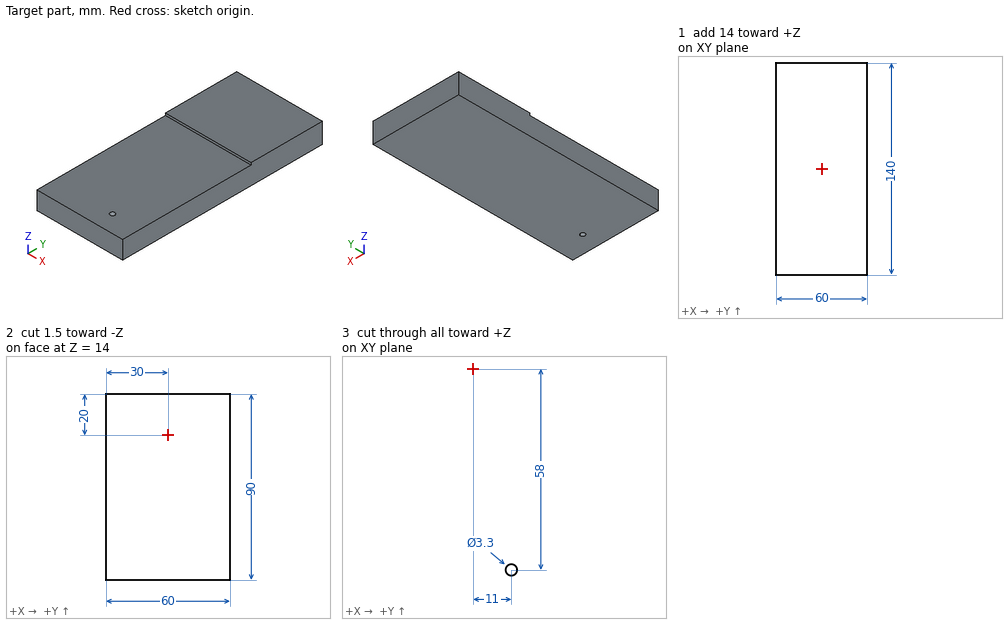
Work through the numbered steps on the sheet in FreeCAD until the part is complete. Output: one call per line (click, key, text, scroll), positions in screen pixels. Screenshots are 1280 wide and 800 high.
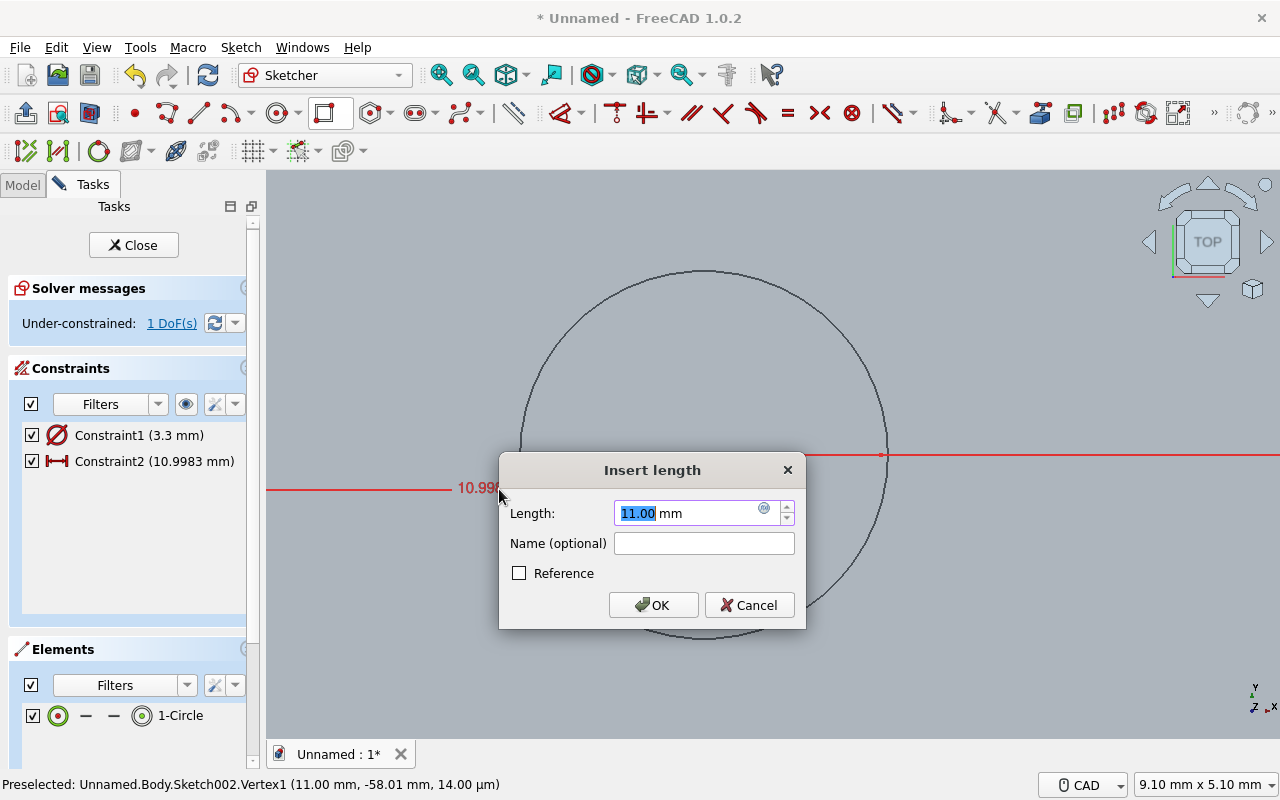
text(11)
key(Return)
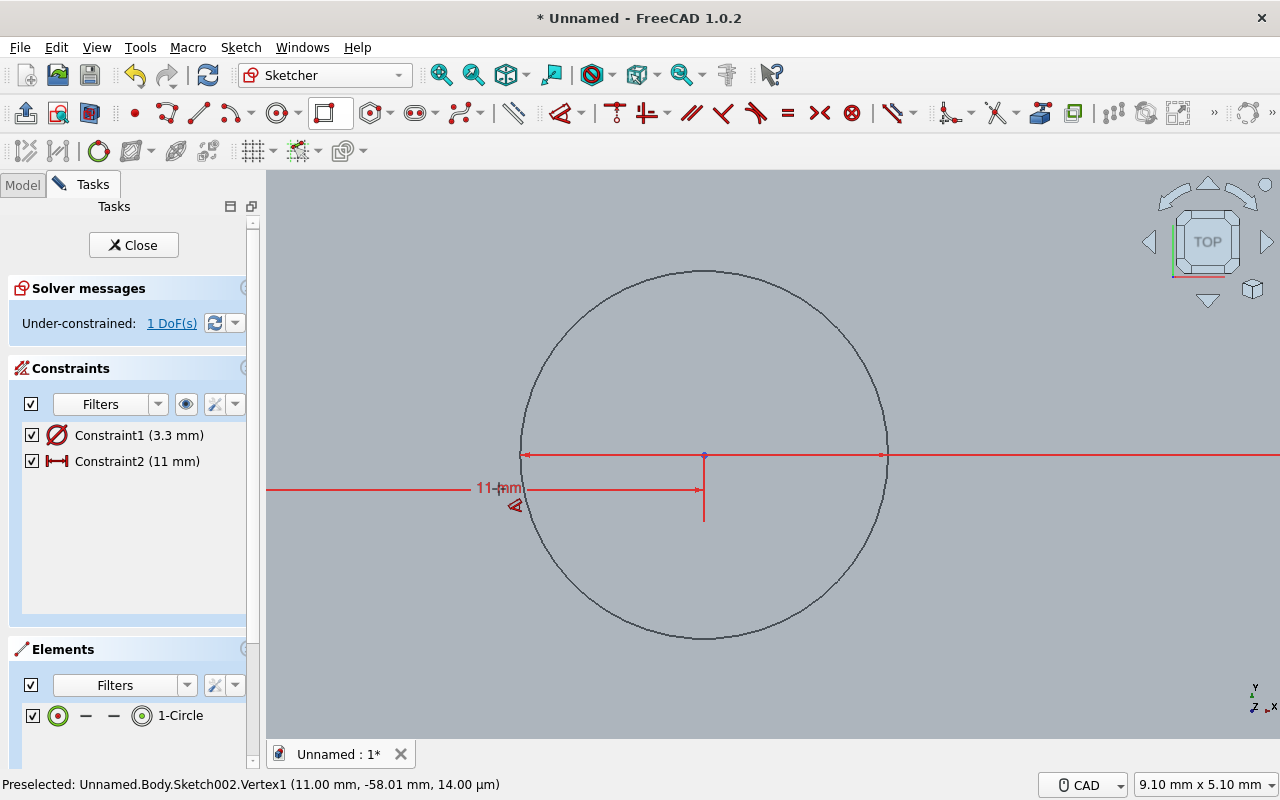
click(704, 455)
click(738, 327)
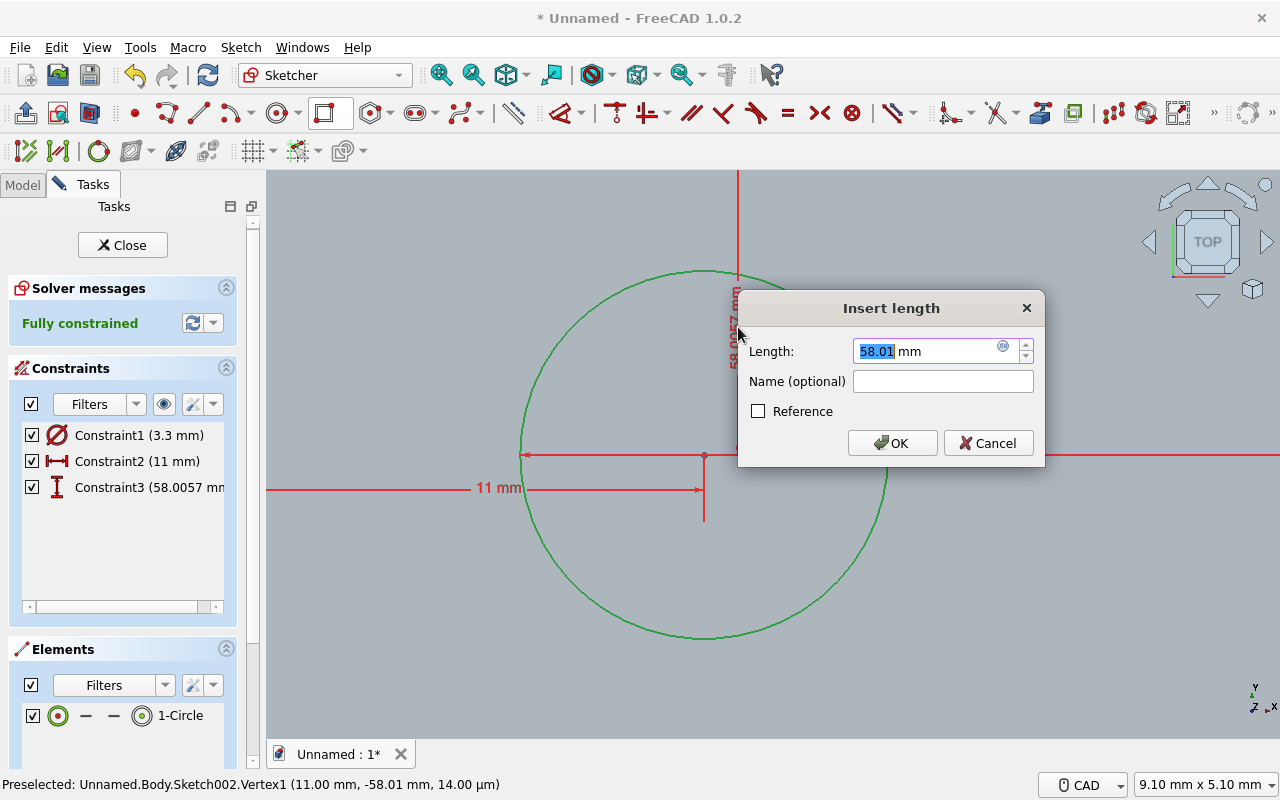
text(58)
key(Return)
key(Escape)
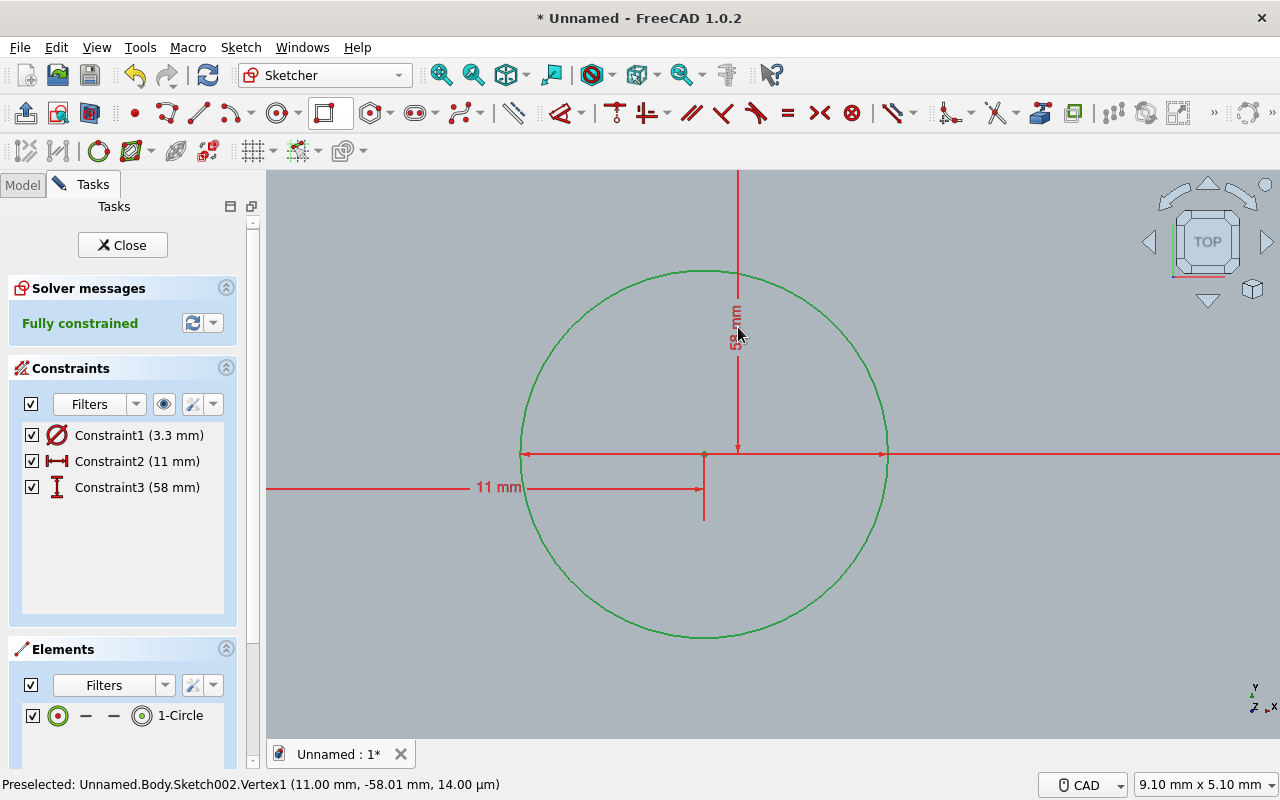
click(123, 245)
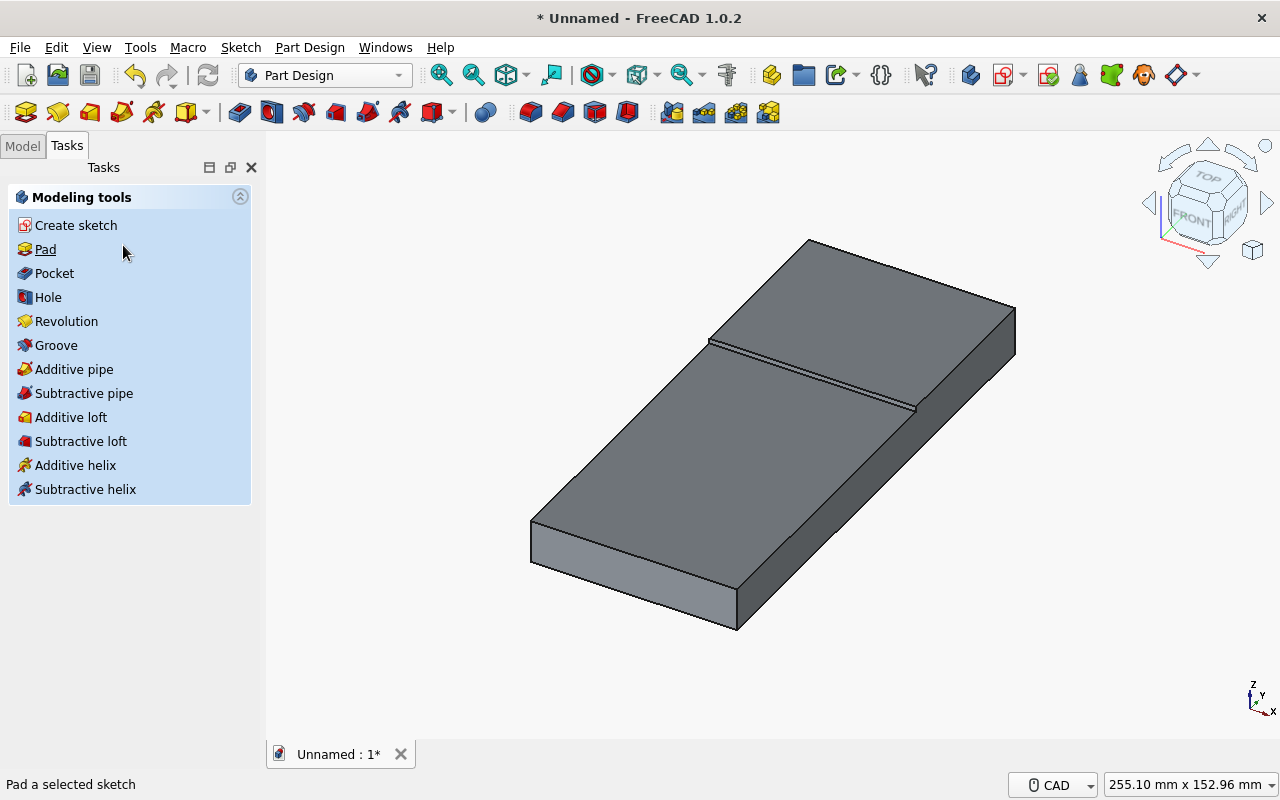
click(240, 112)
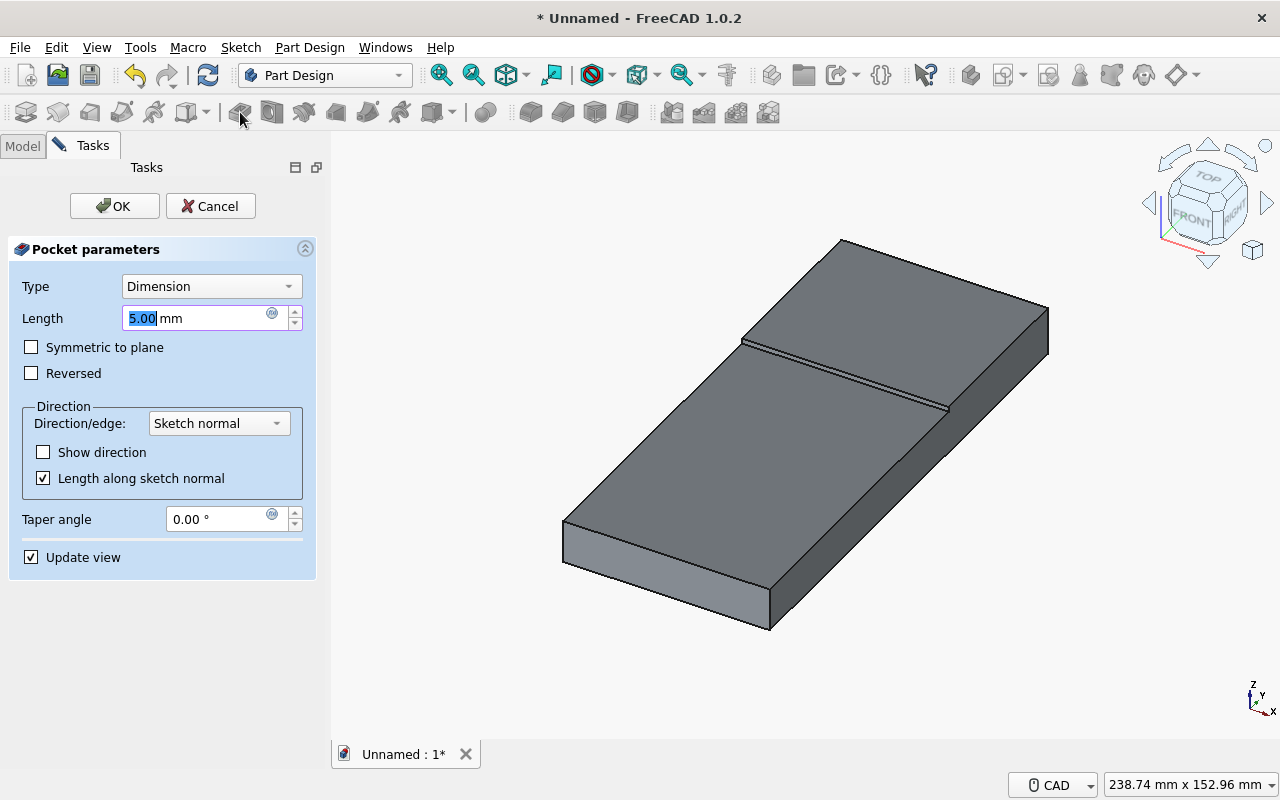
click(212, 286)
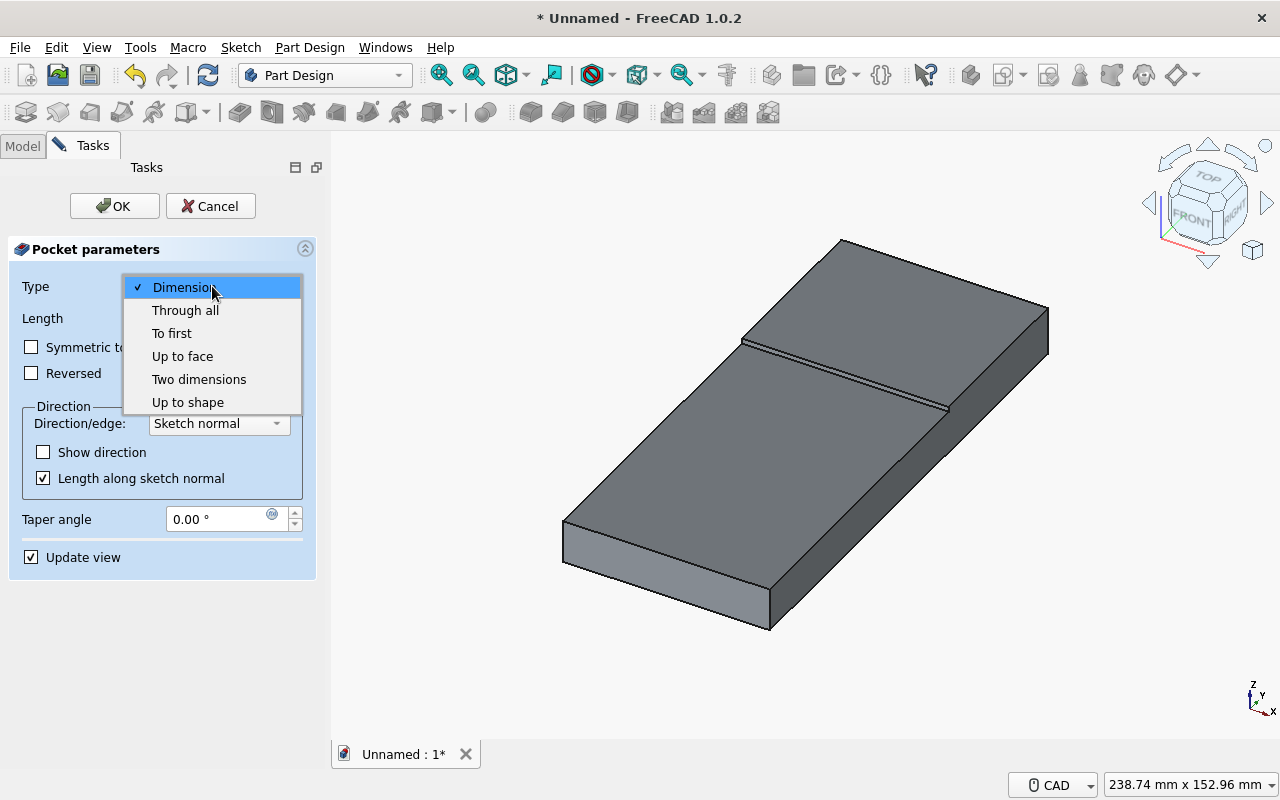
click(212, 310)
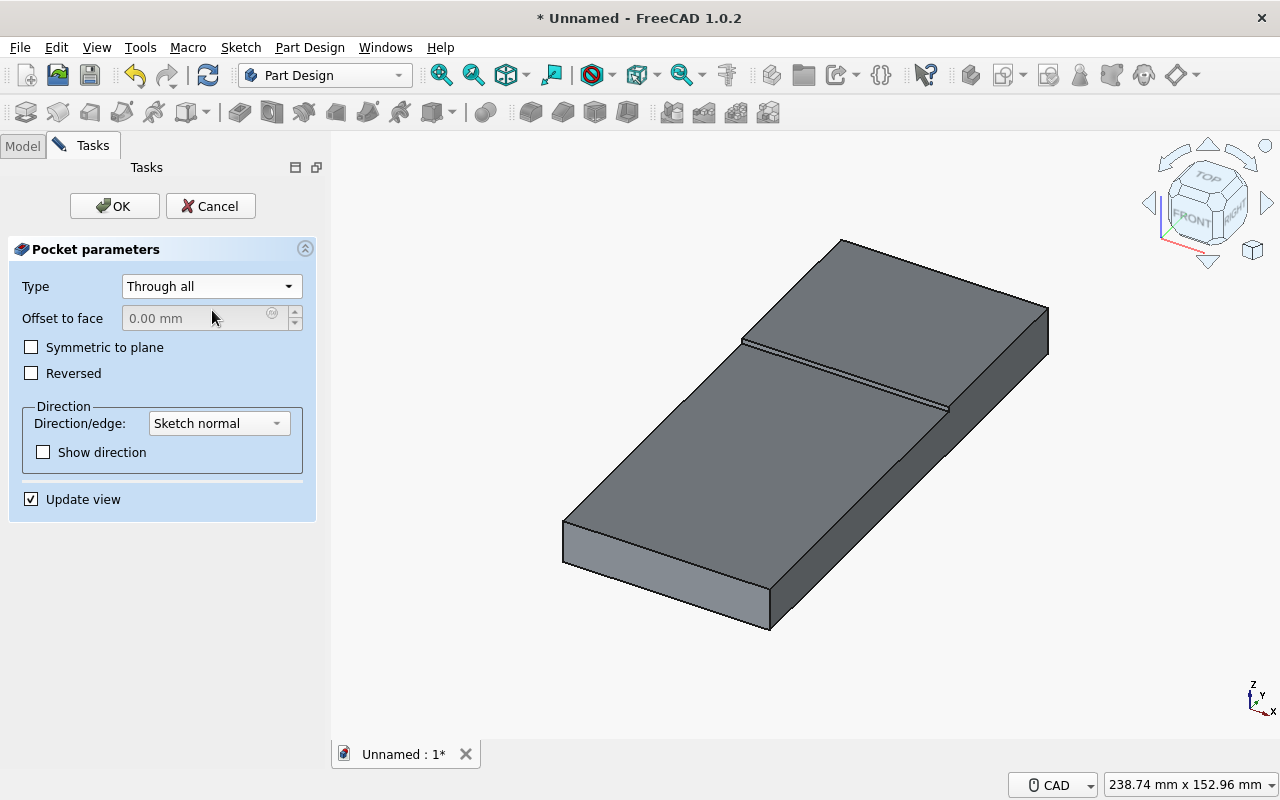
click(30, 373)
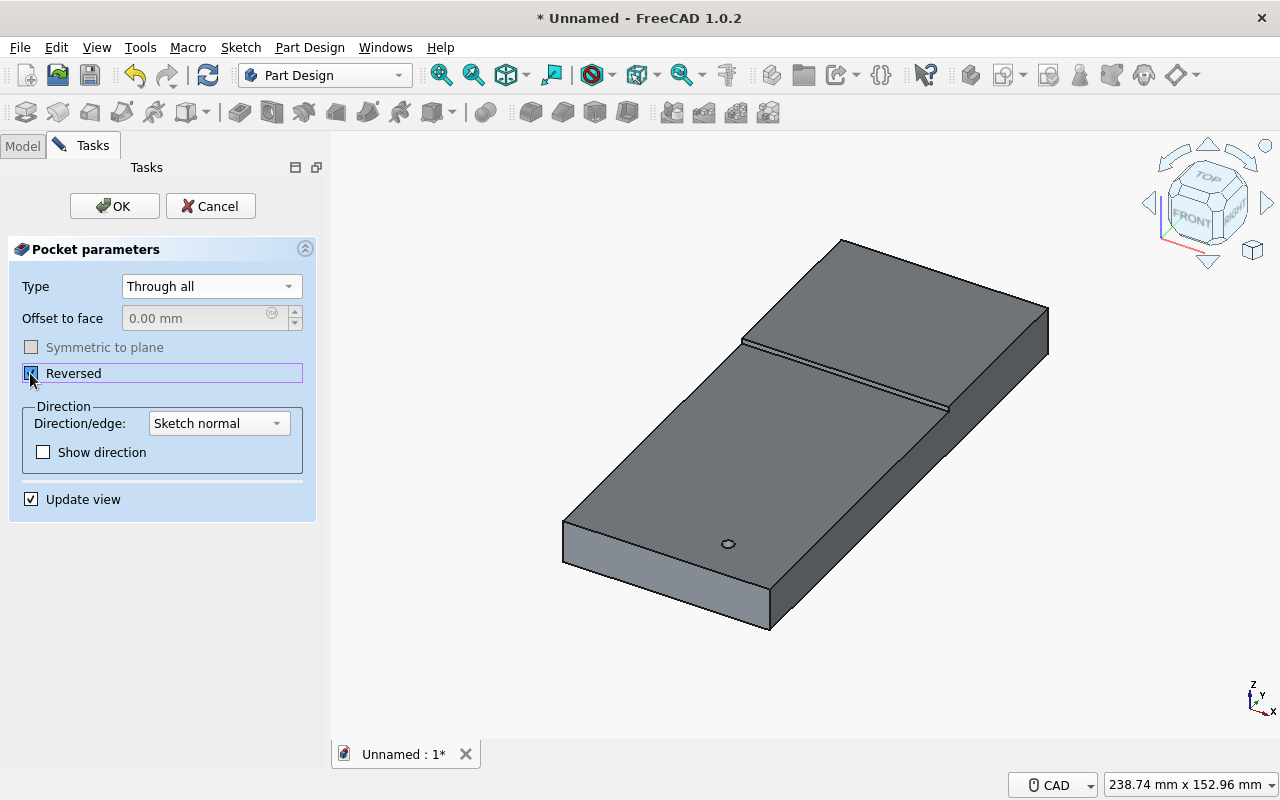
click(115, 206)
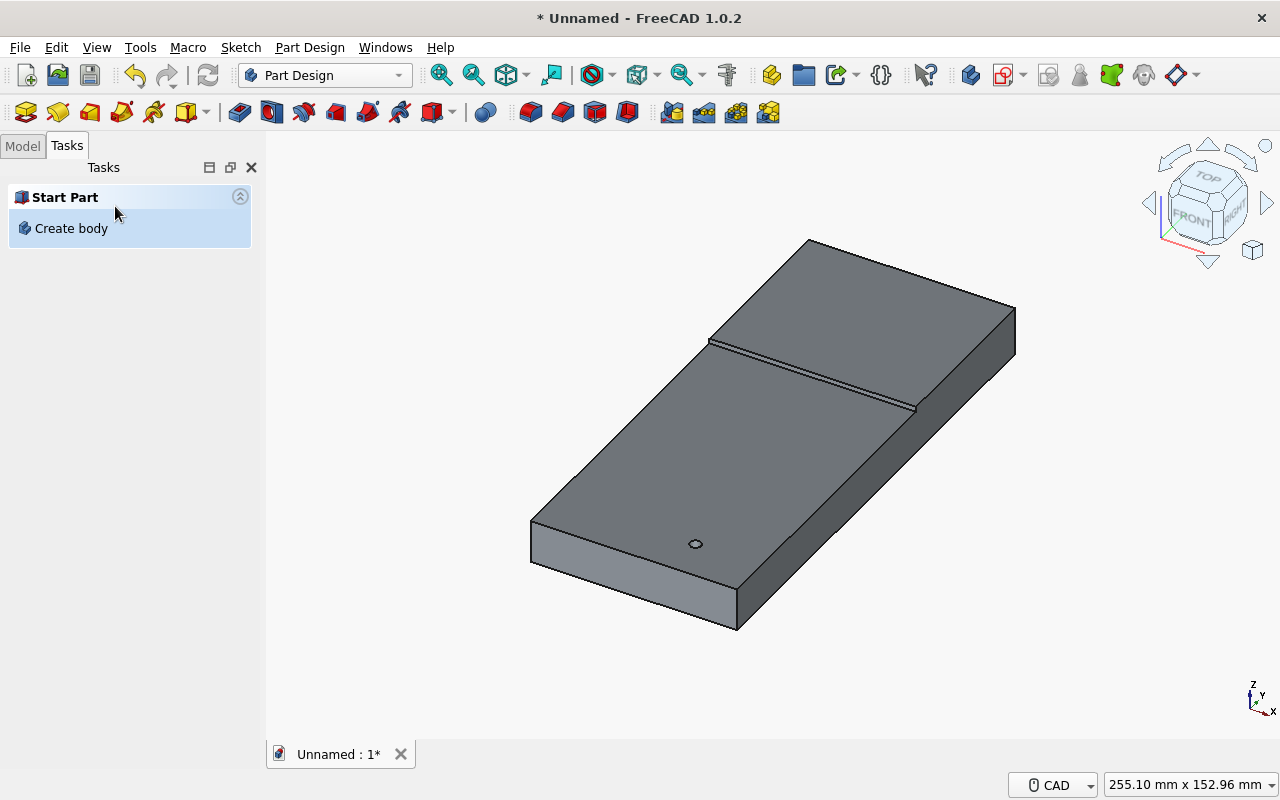
key(0)